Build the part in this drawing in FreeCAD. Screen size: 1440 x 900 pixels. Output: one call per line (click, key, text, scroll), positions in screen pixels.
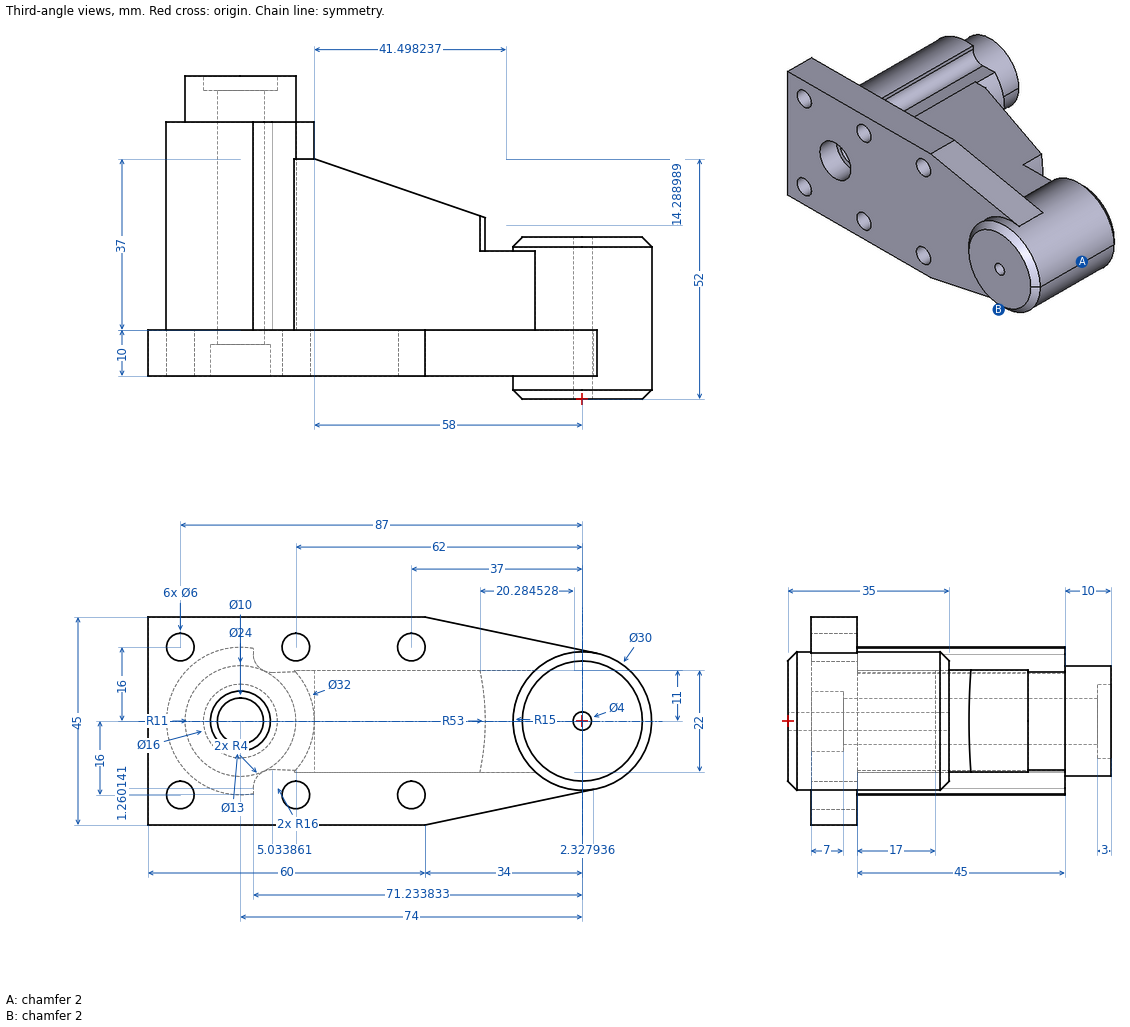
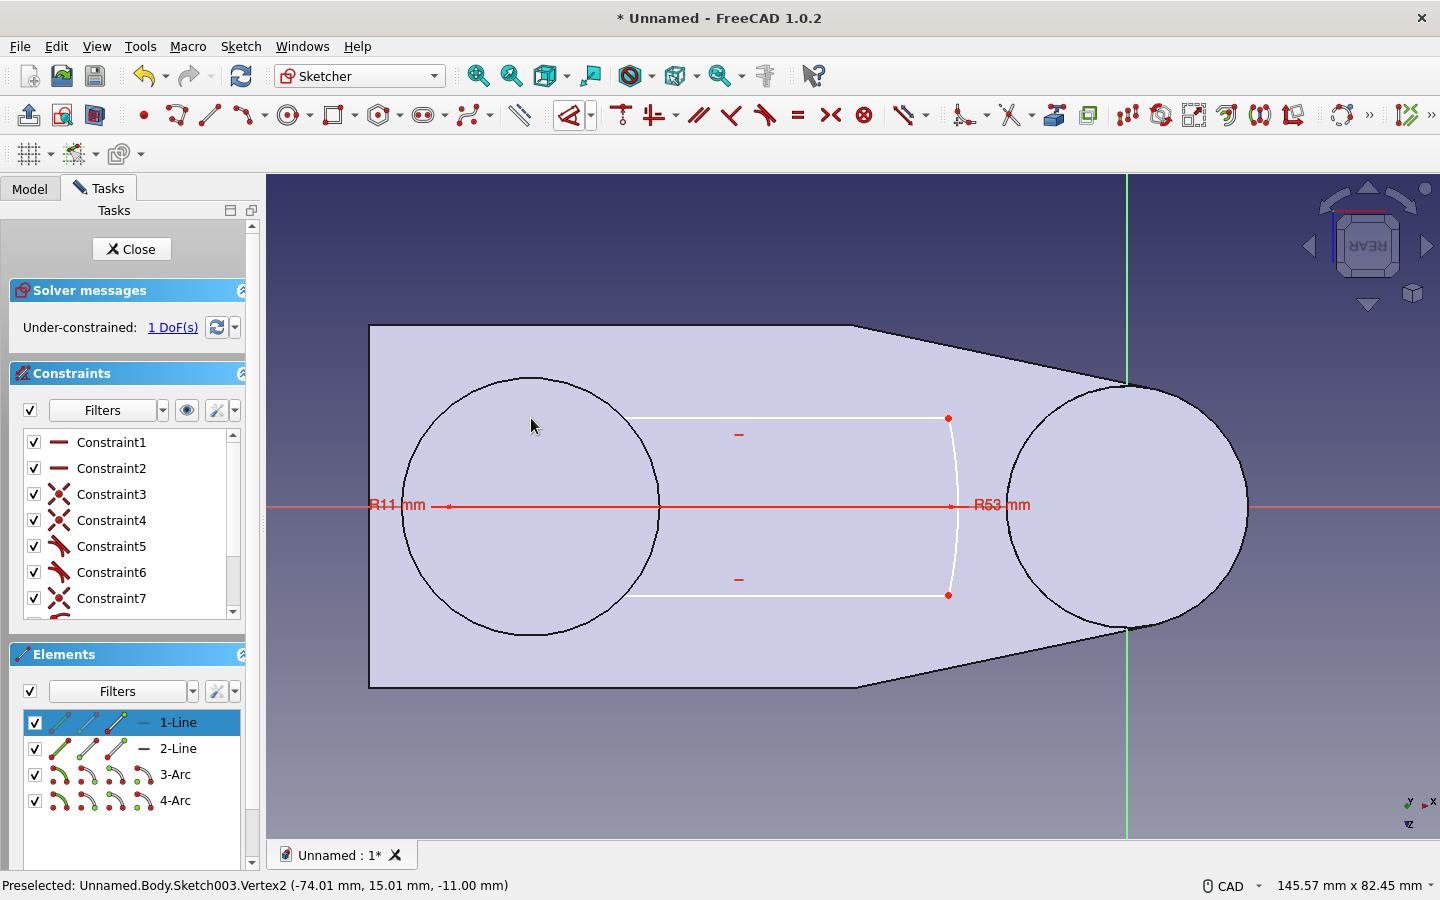
click(590, 116)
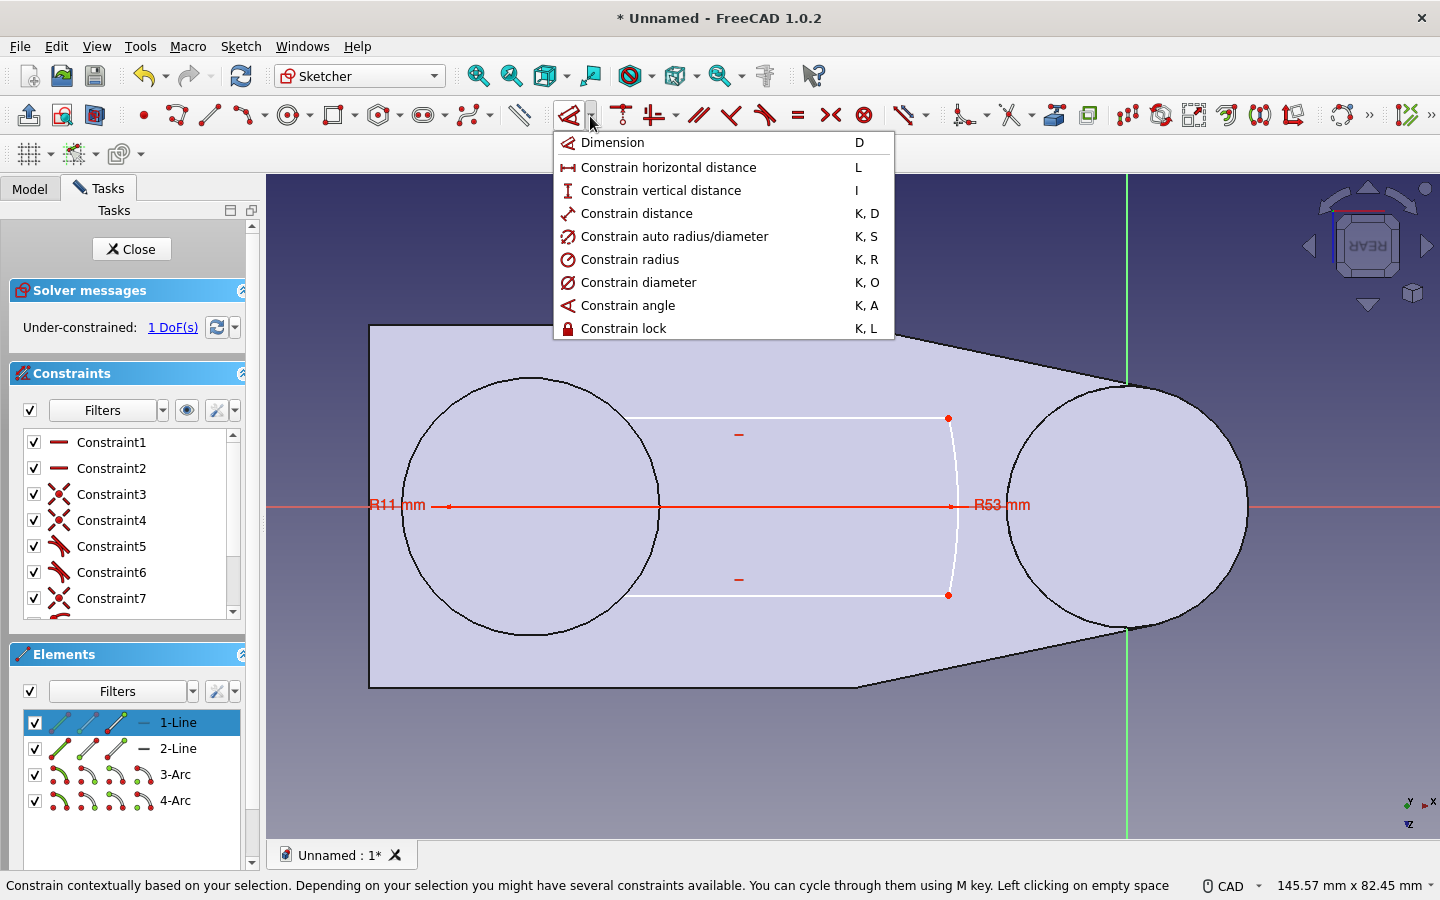
click(724, 168)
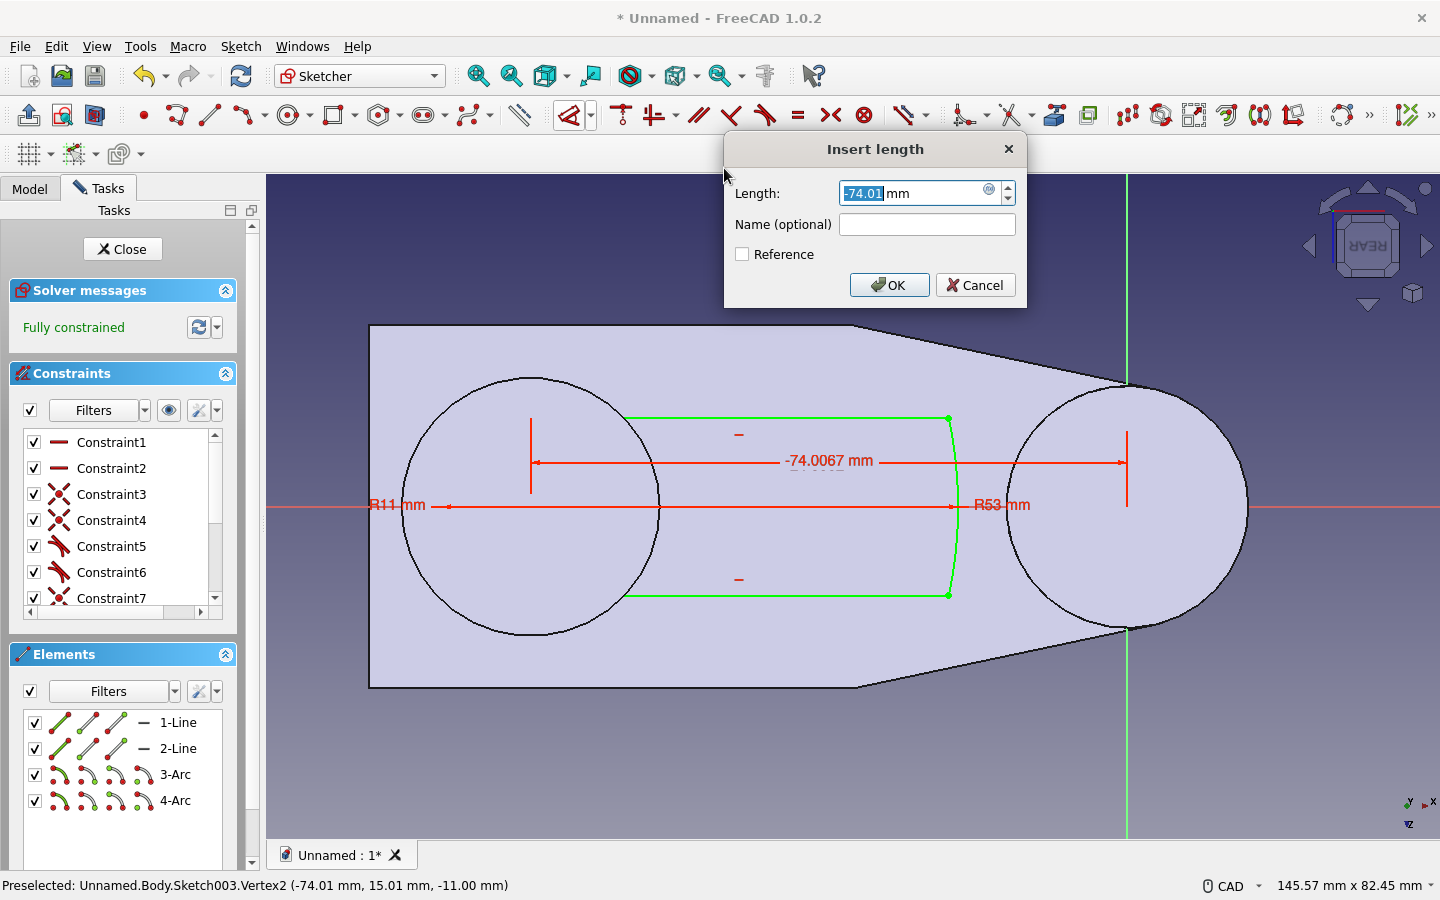
text(-74)
key(Return)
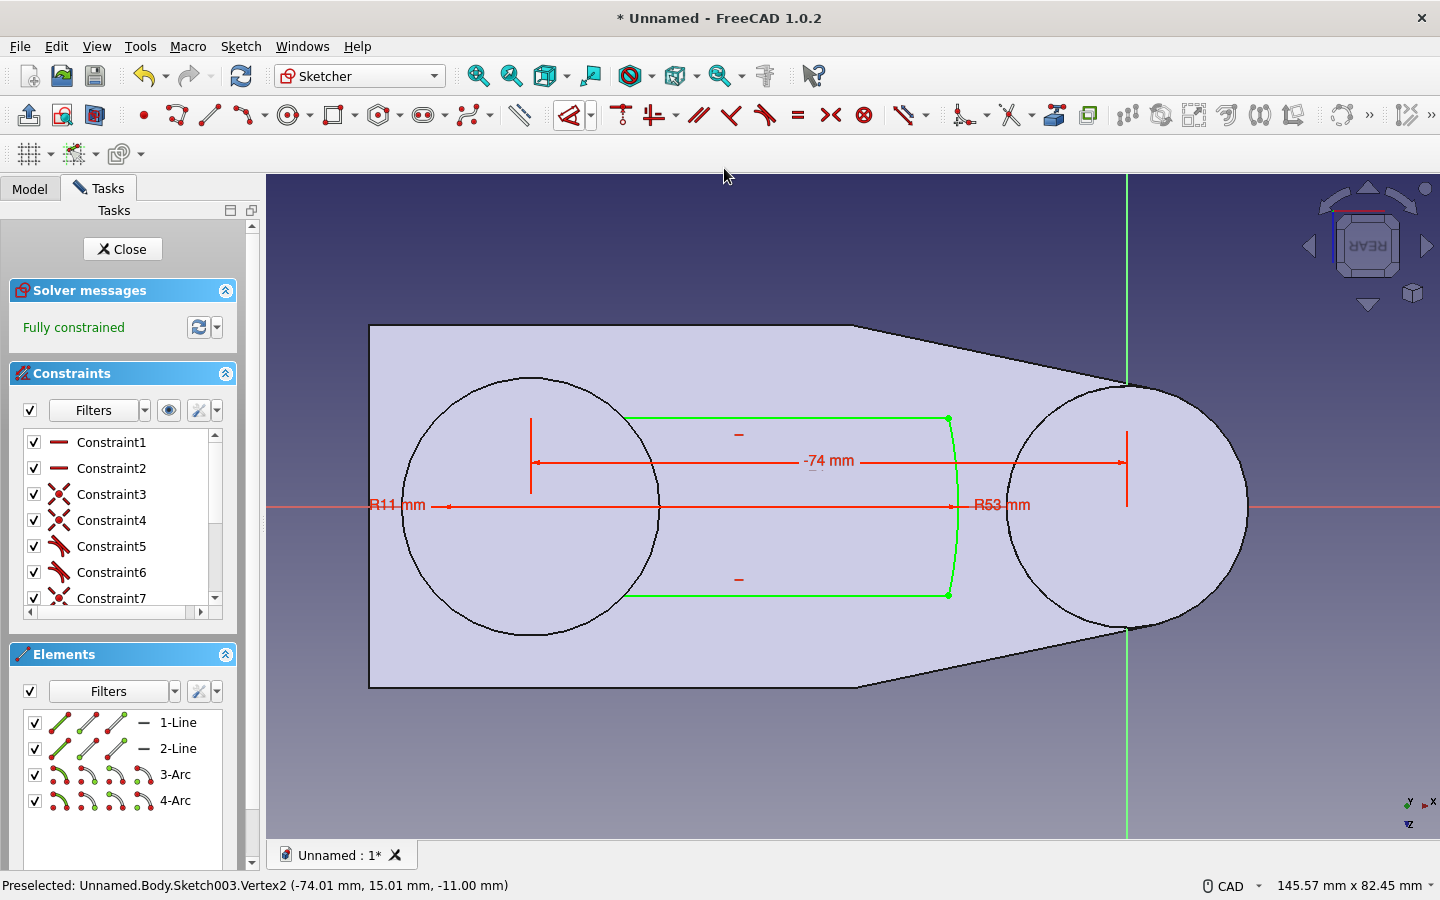
click(123, 249)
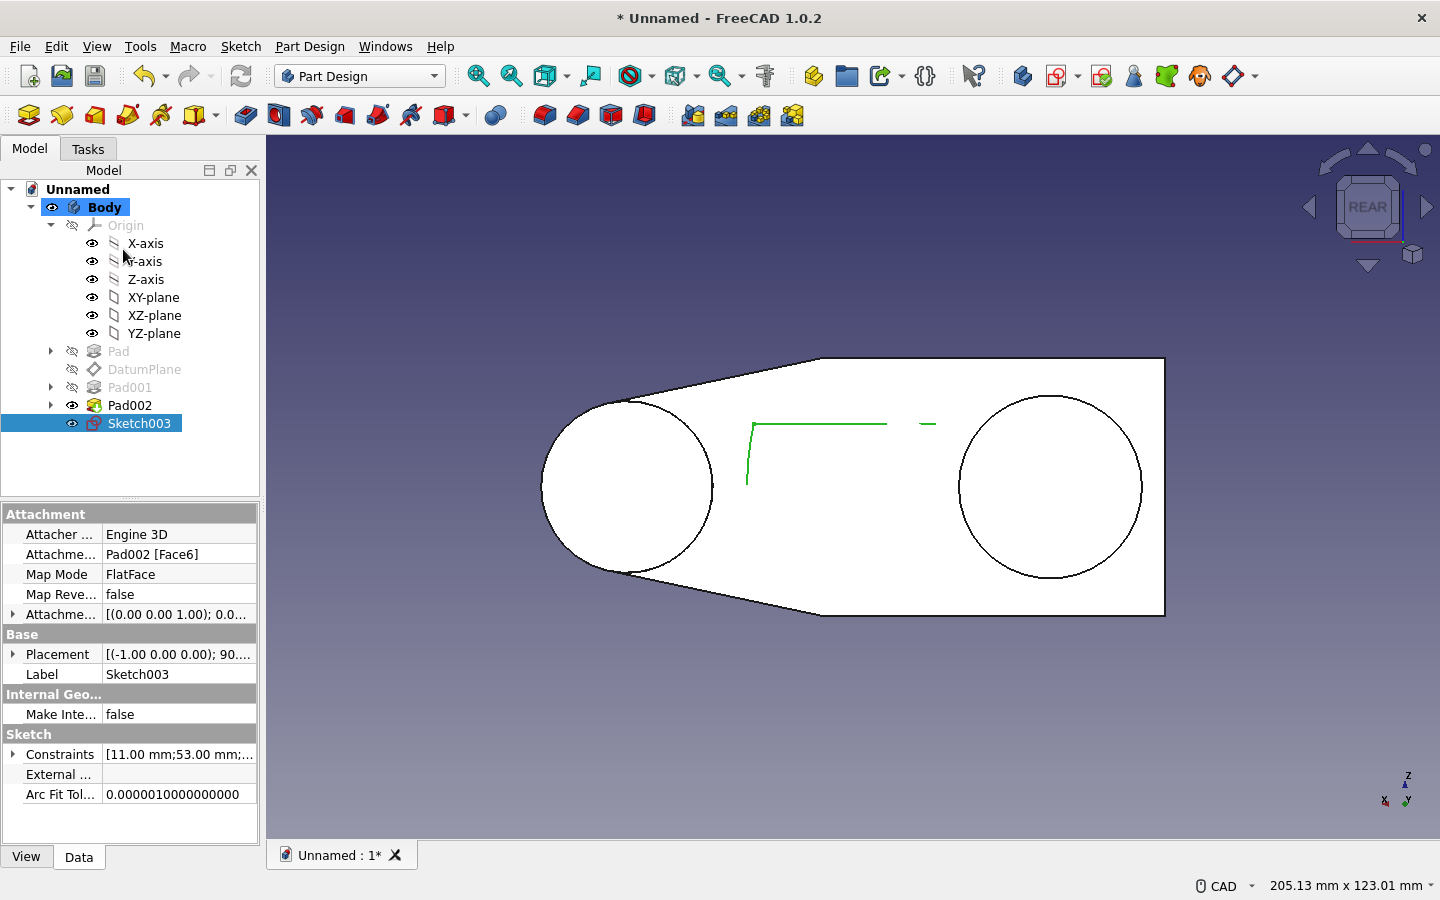
click(29, 116)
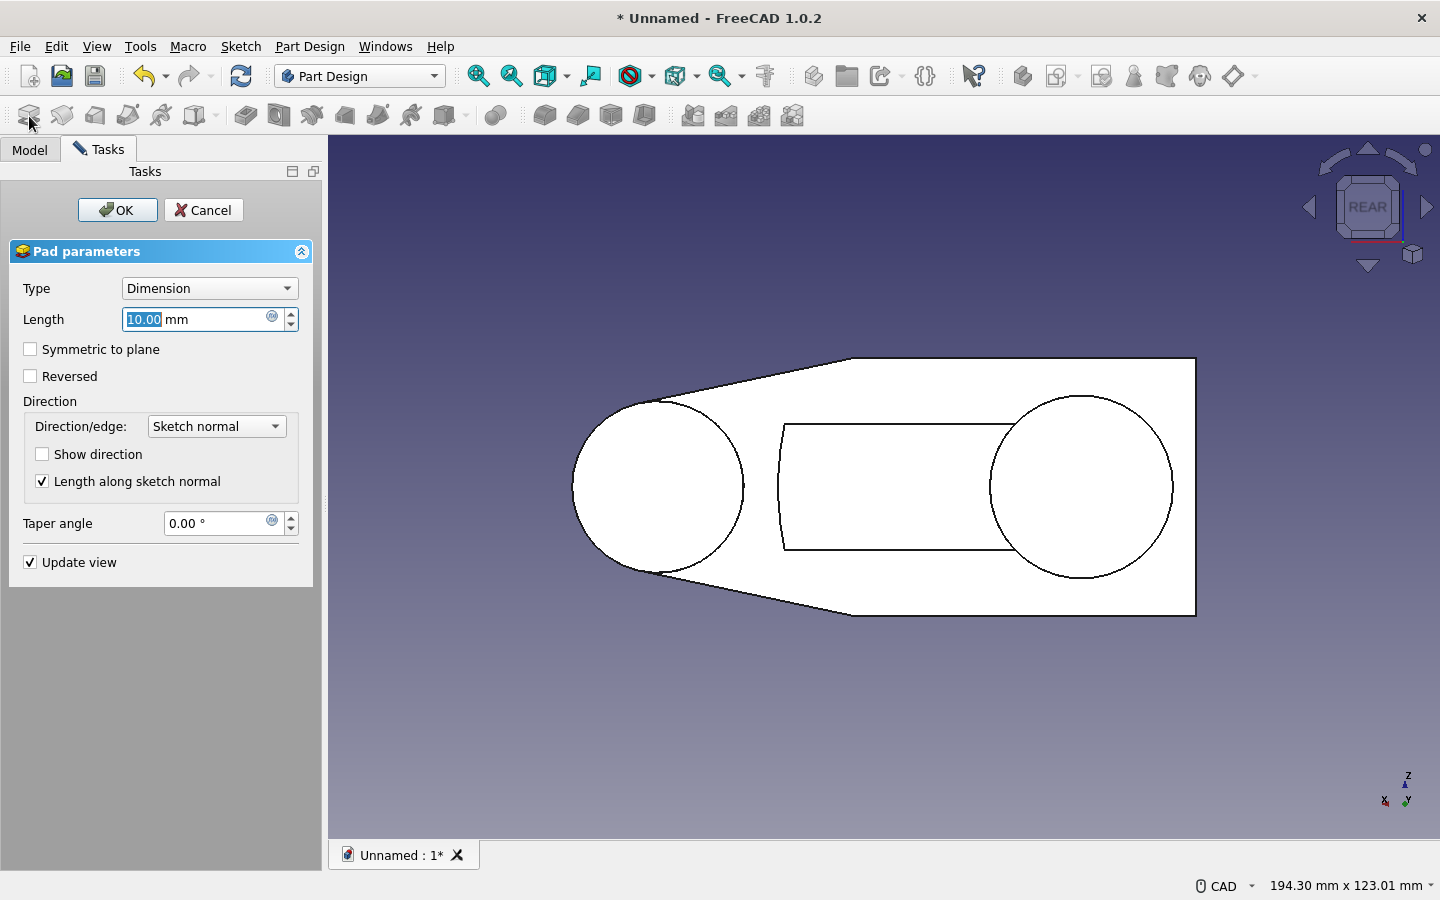
text(37)
key(Tab)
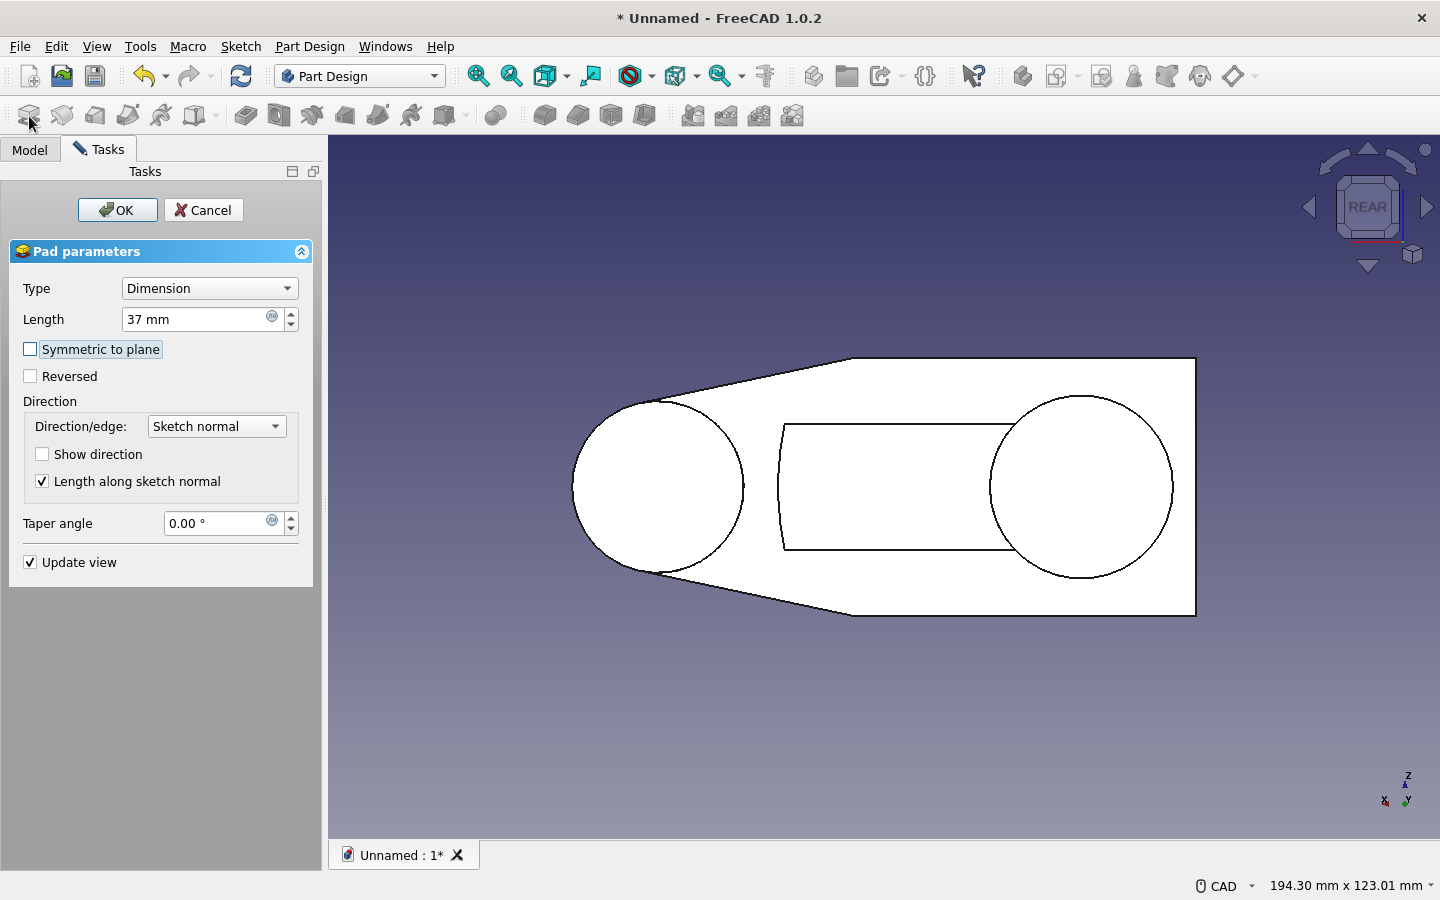
click(118, 210)